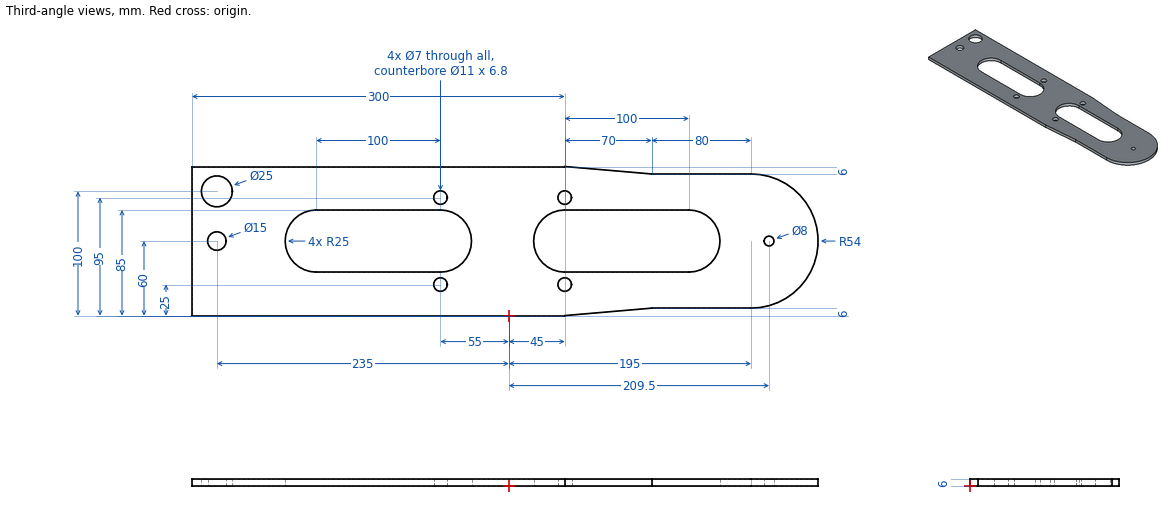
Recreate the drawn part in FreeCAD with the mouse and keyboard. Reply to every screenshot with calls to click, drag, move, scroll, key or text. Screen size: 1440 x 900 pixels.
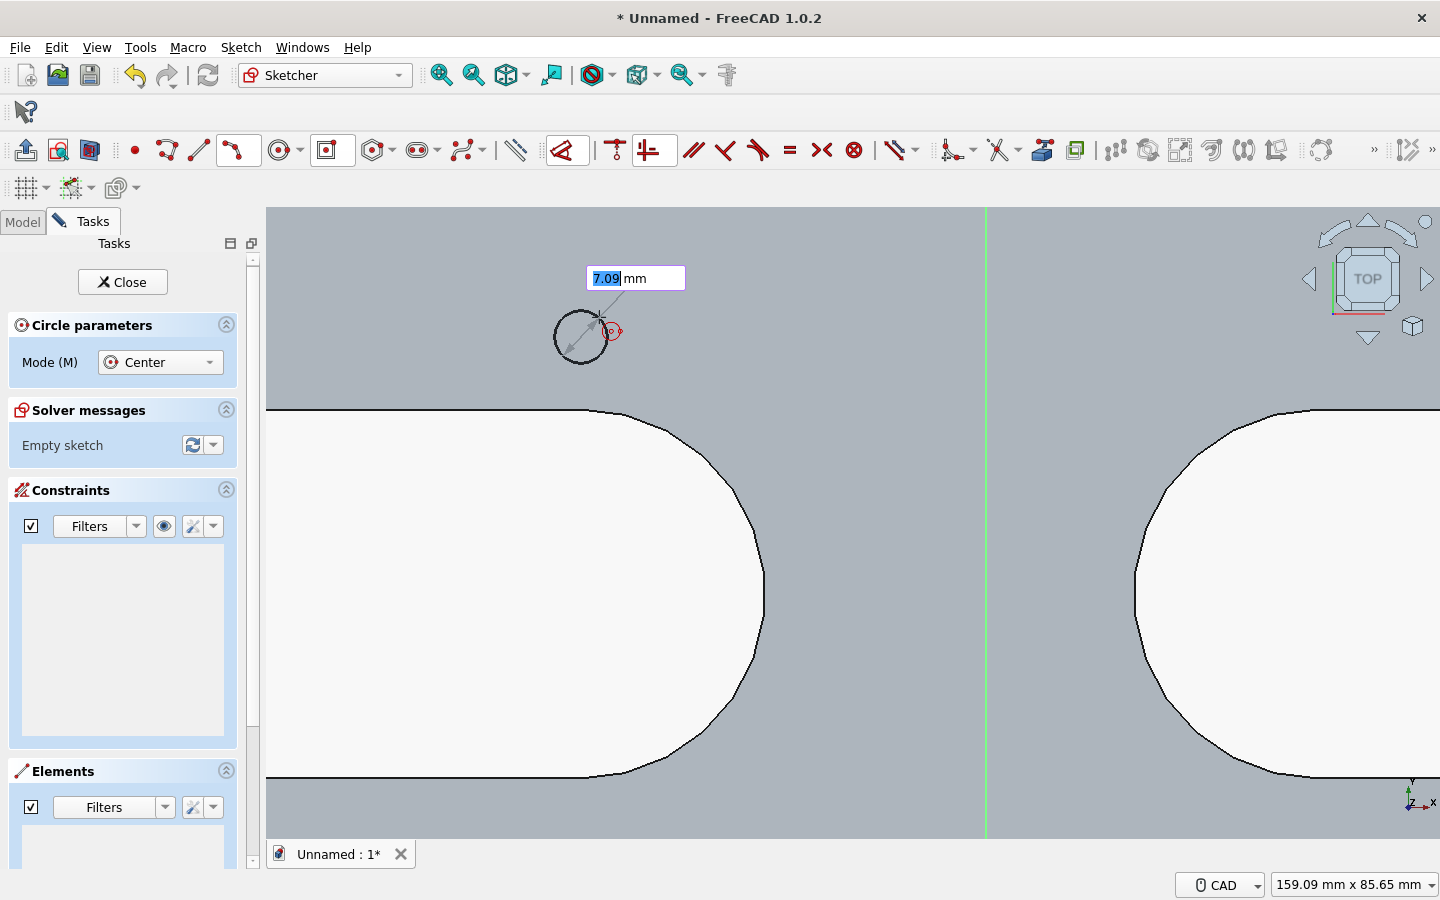
text(7)
key(Return)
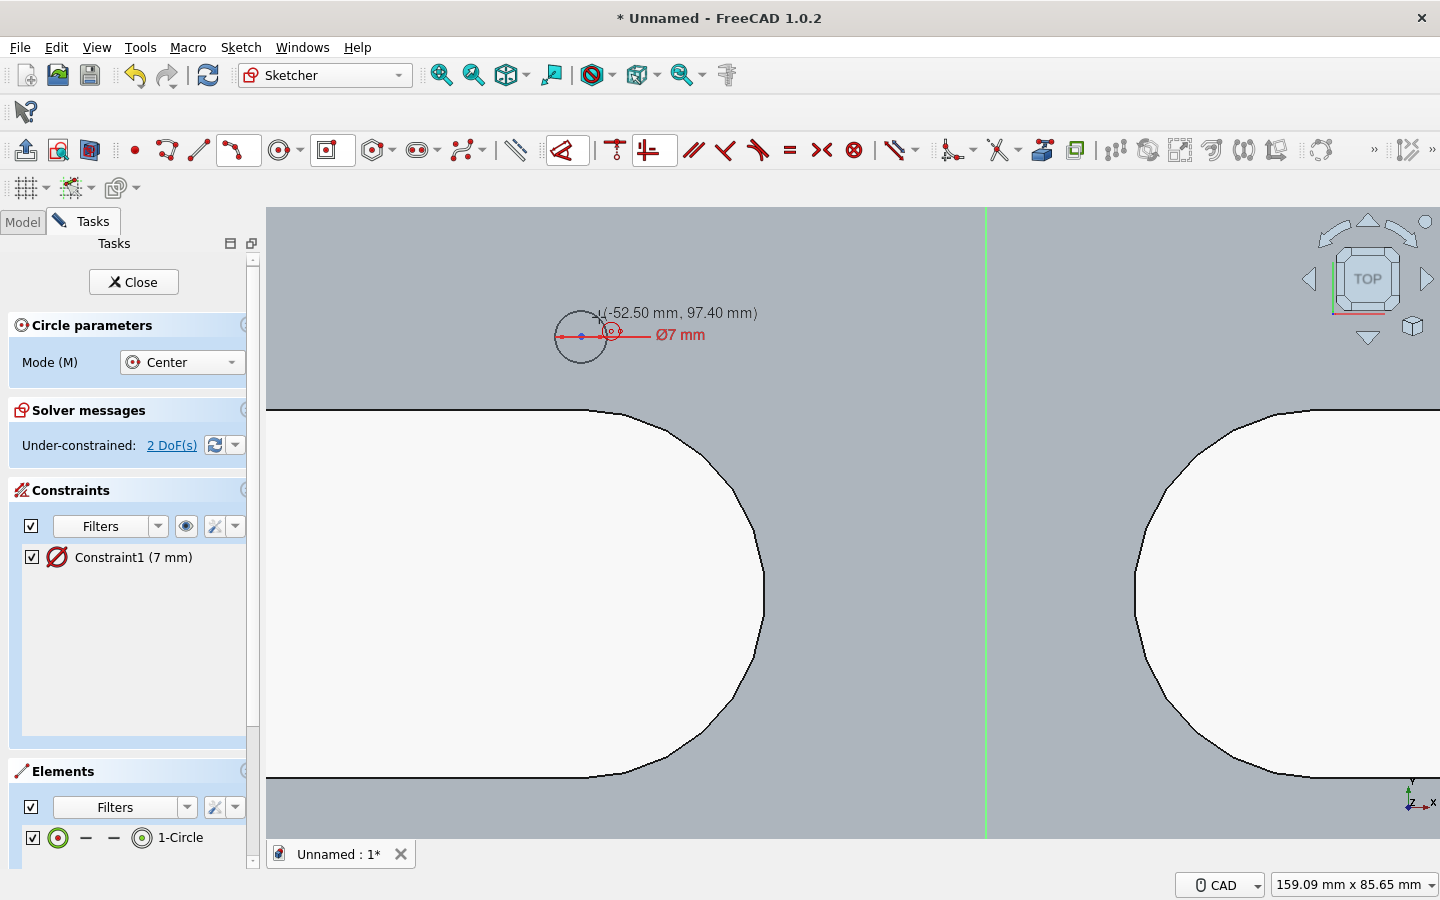
scroll(584, 340, down, 3)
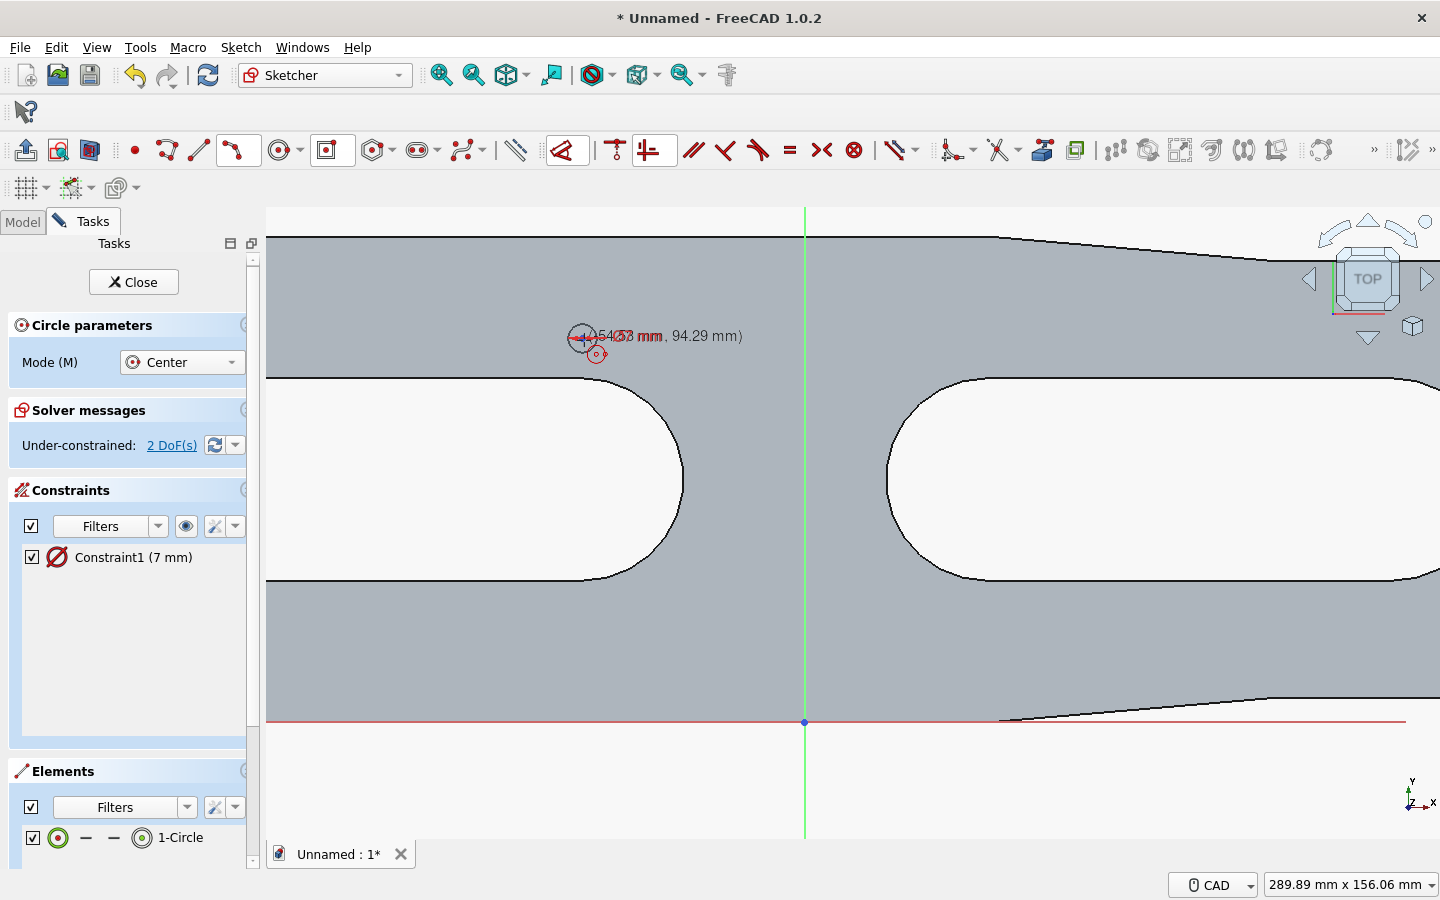
scroll(582, 621, up, 3)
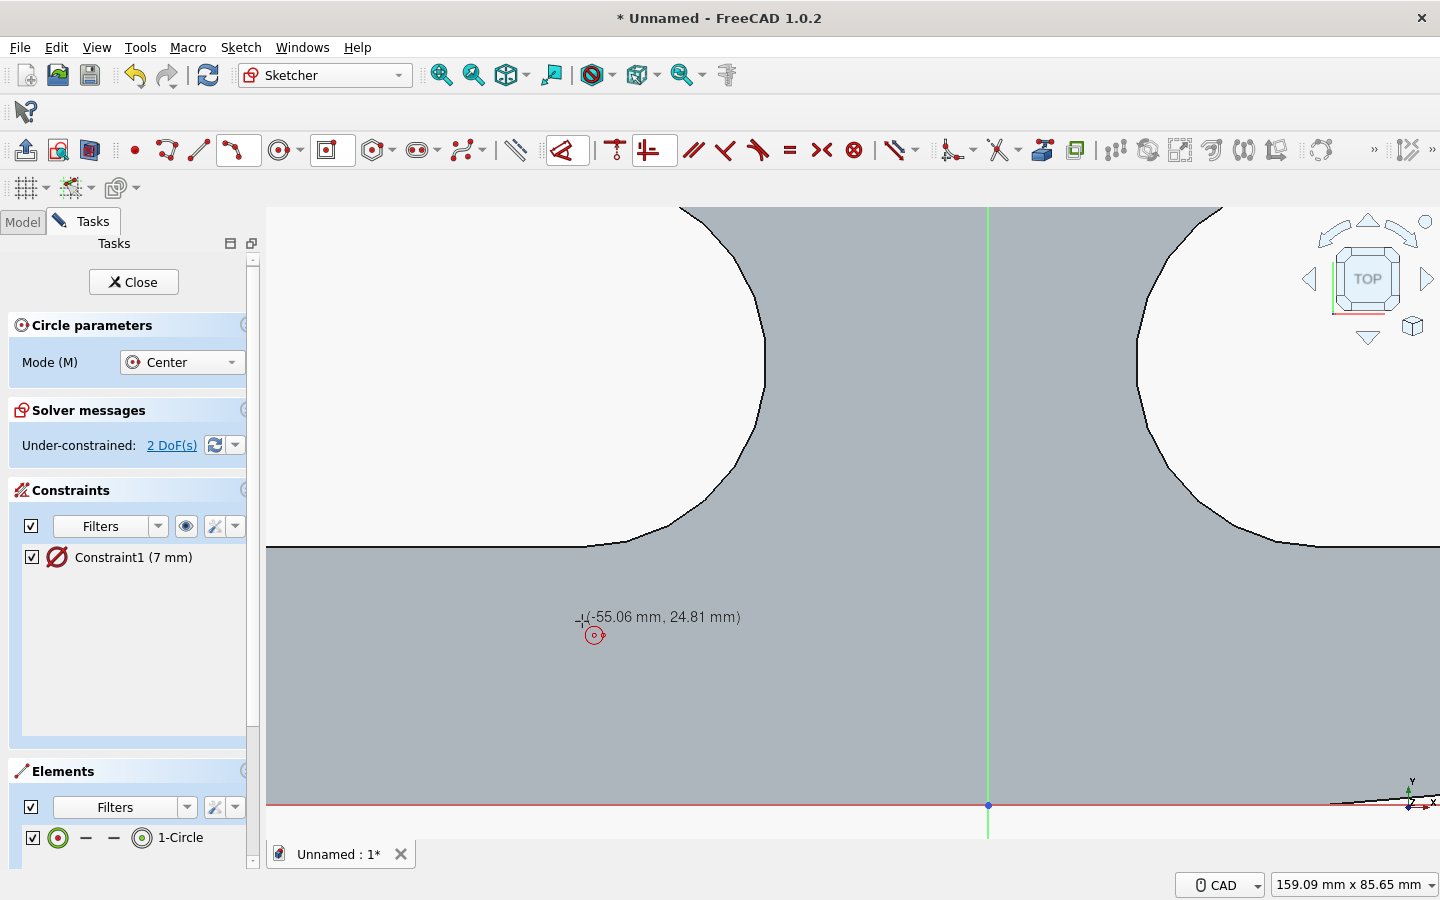
click(582, 621)
move(600, 603)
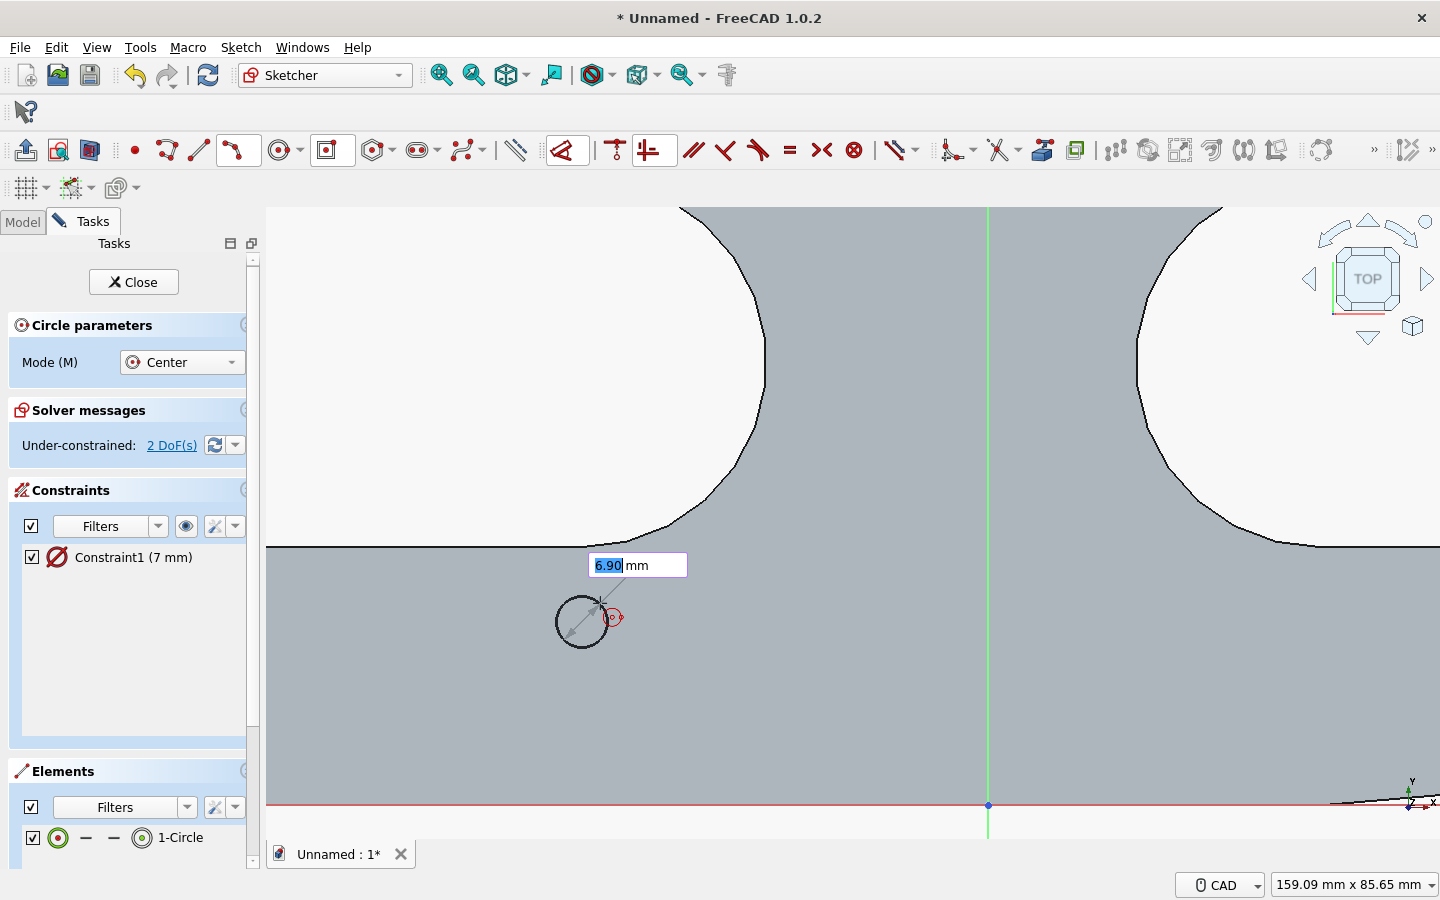
text(7)
key(Return)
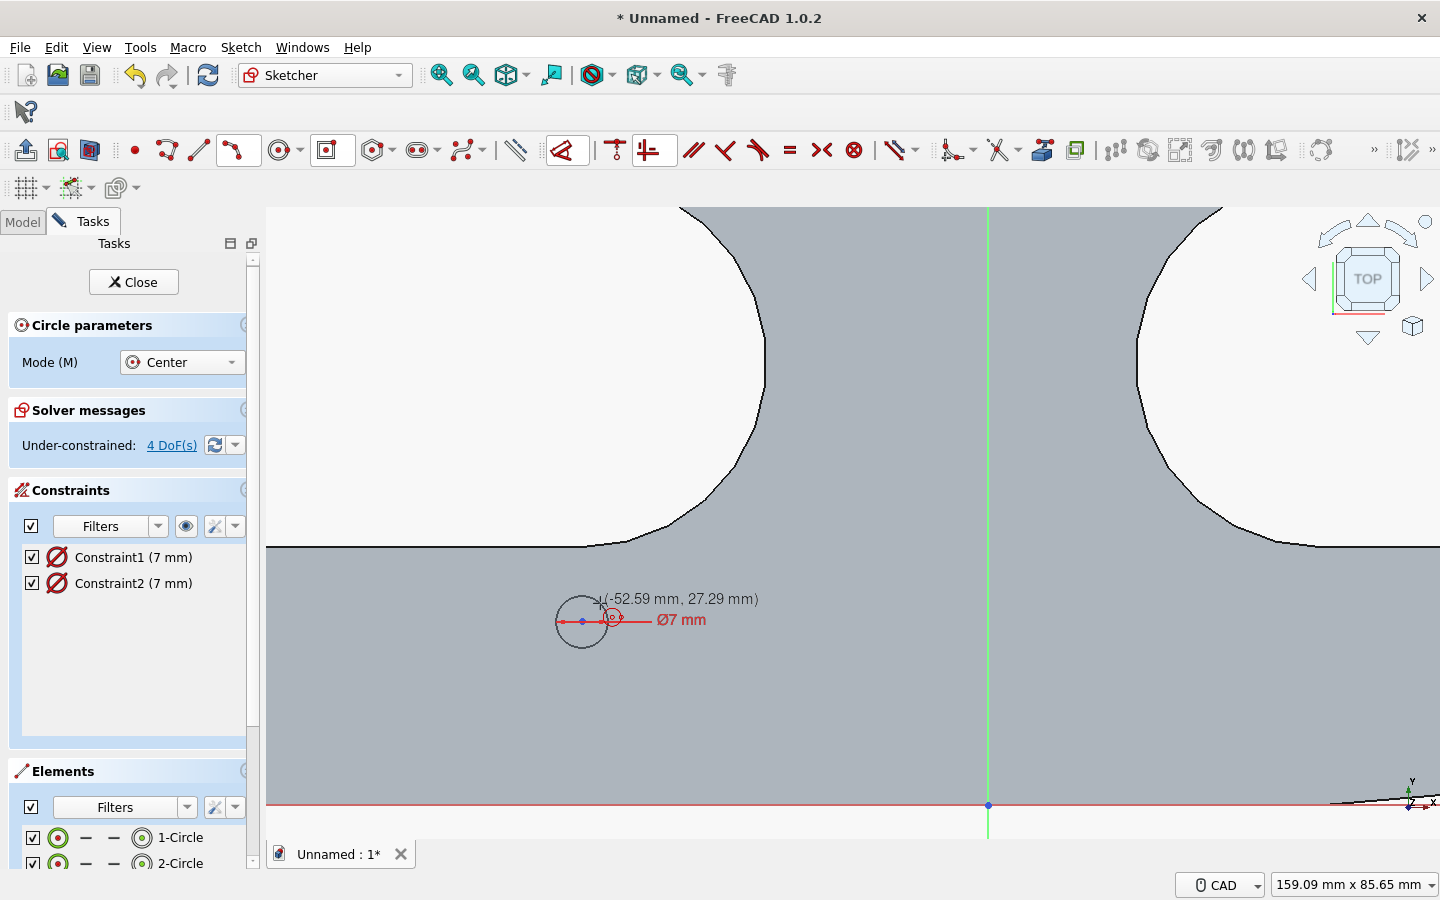
scroll(582, 622, down, 3)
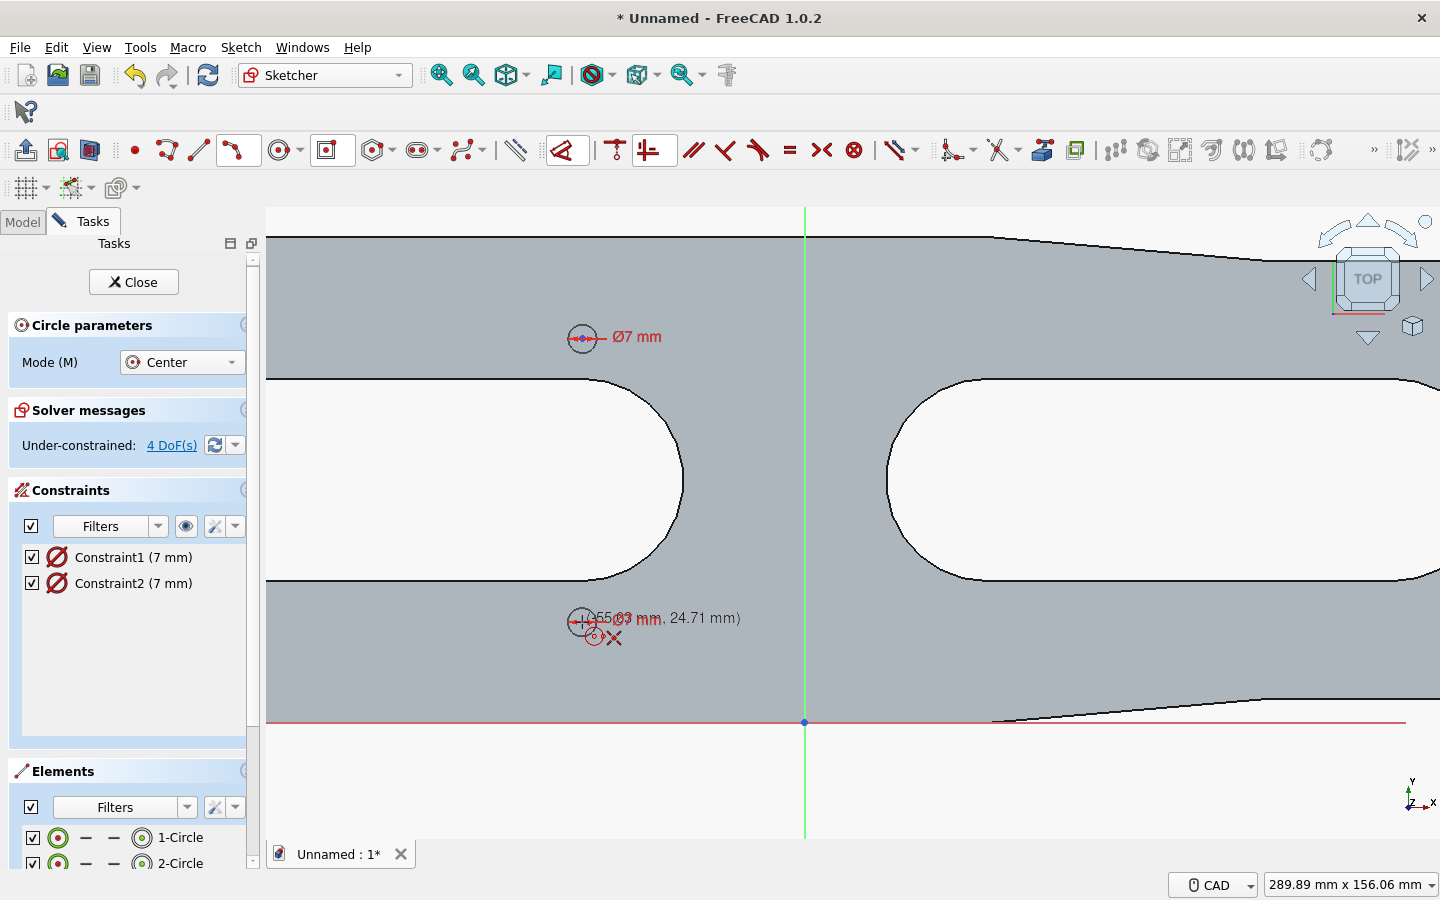
scroll(987, 338, up, 3)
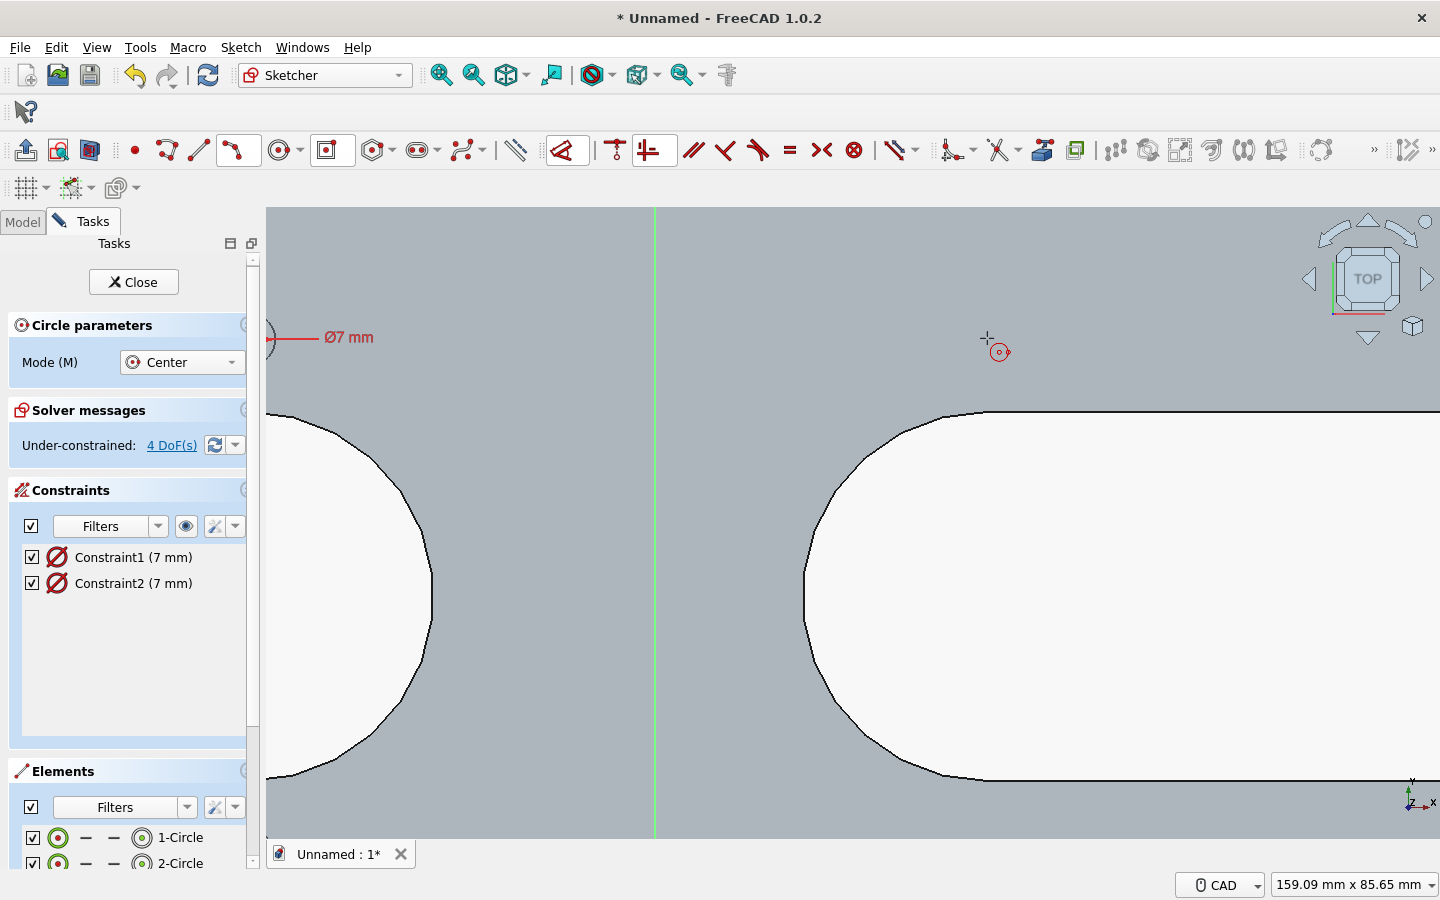
click(987, 338)
move(1005, 320)